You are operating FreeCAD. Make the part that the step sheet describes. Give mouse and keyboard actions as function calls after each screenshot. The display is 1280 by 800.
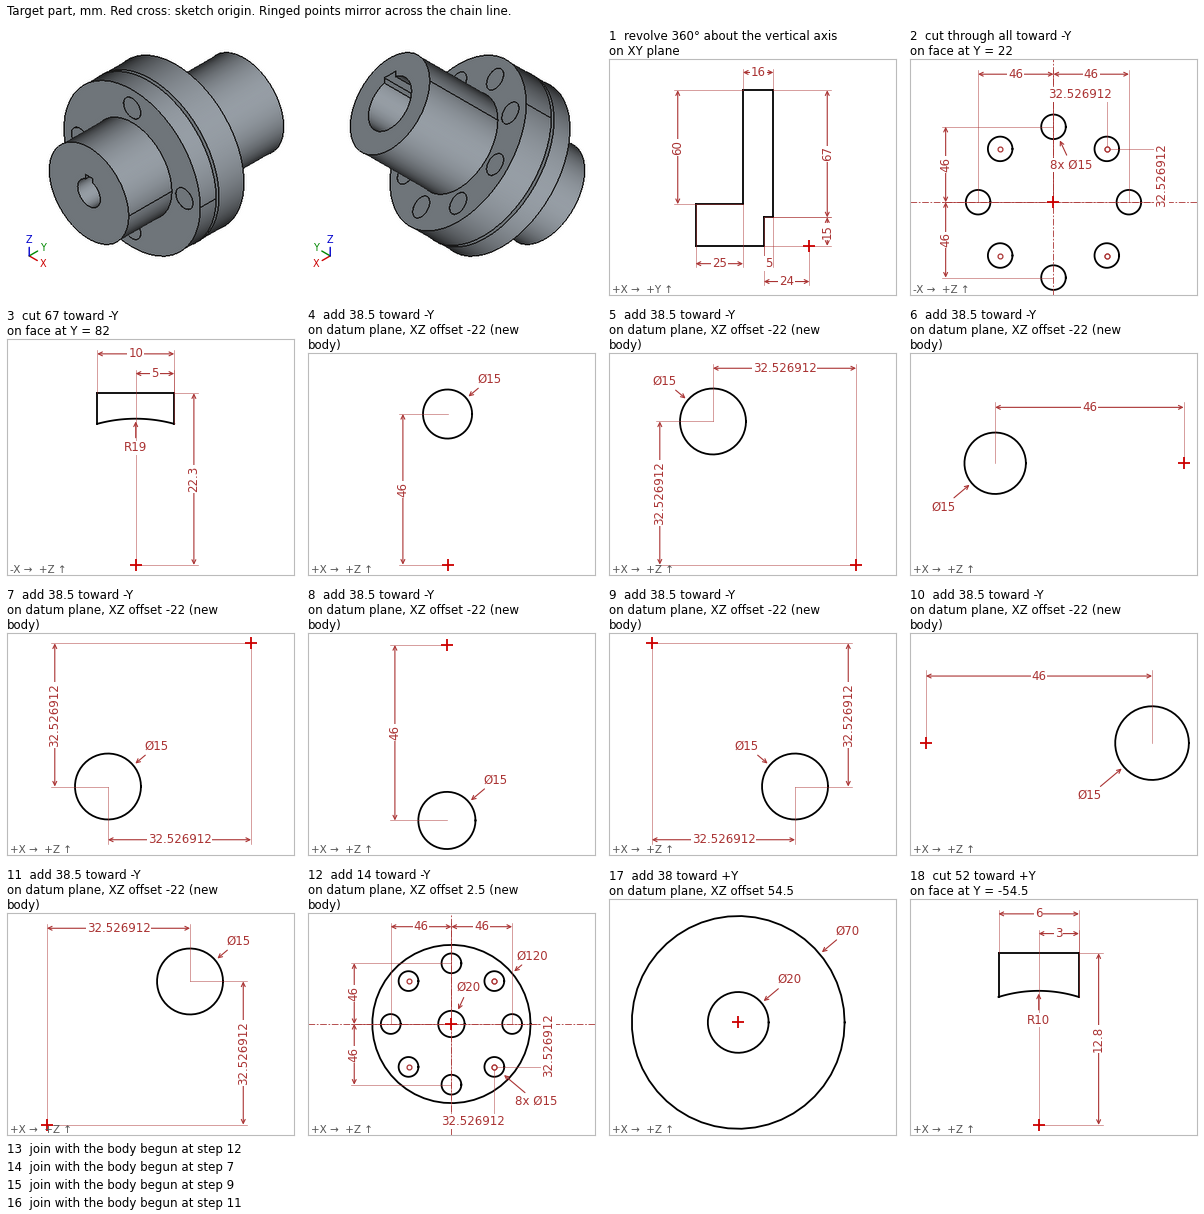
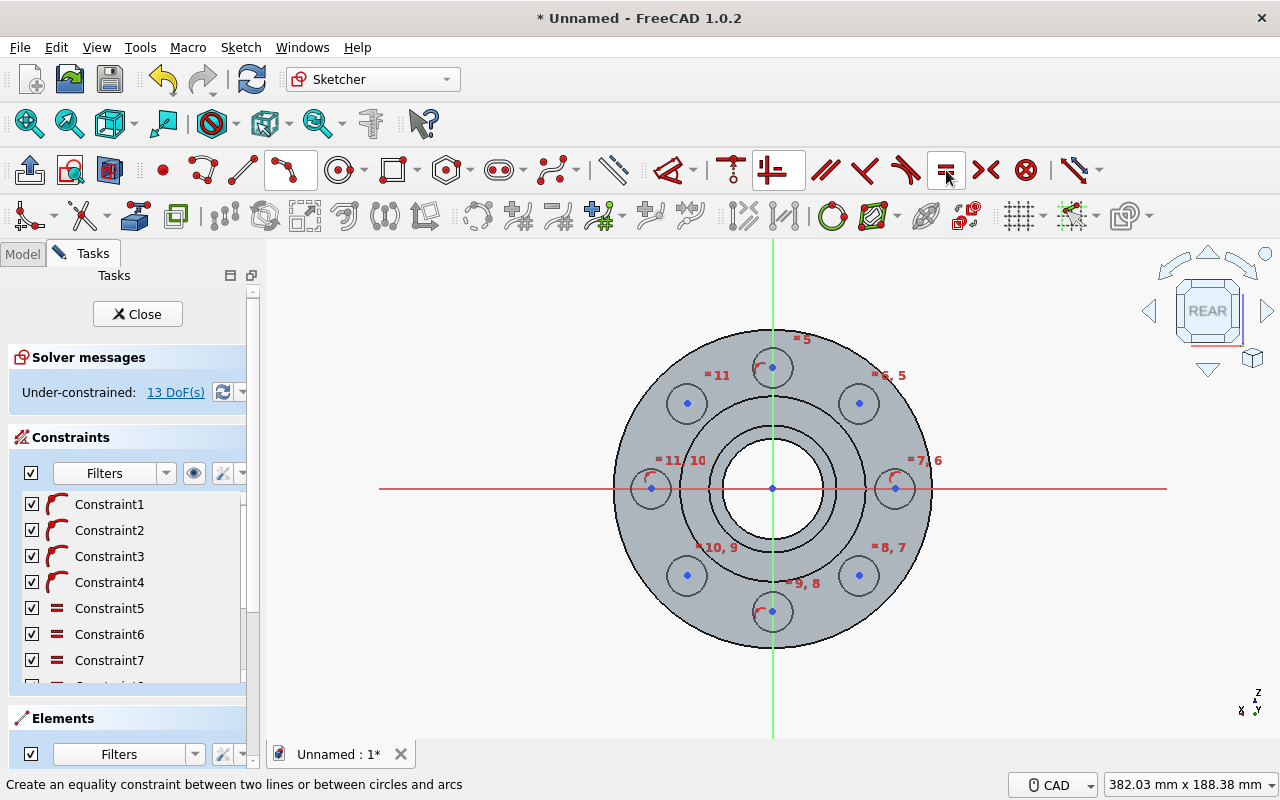
click(859, 404)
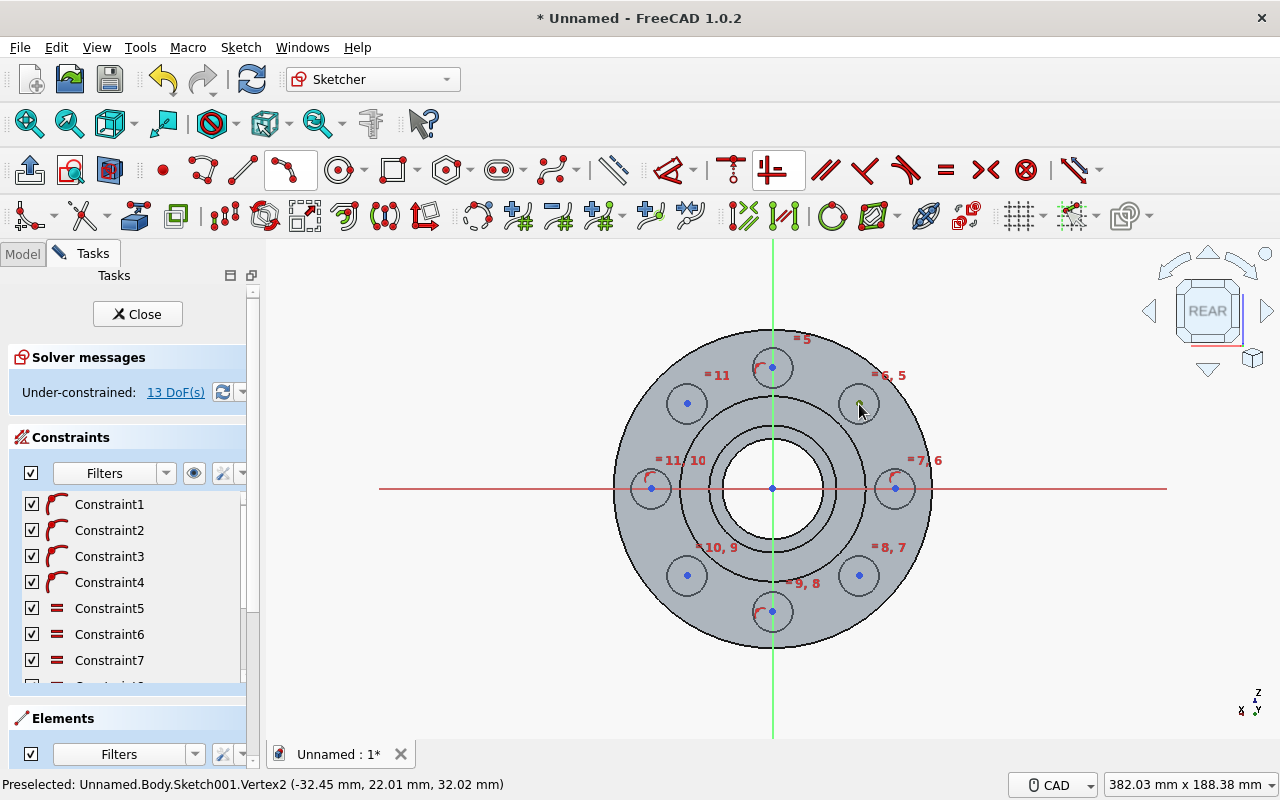
click(859, 576)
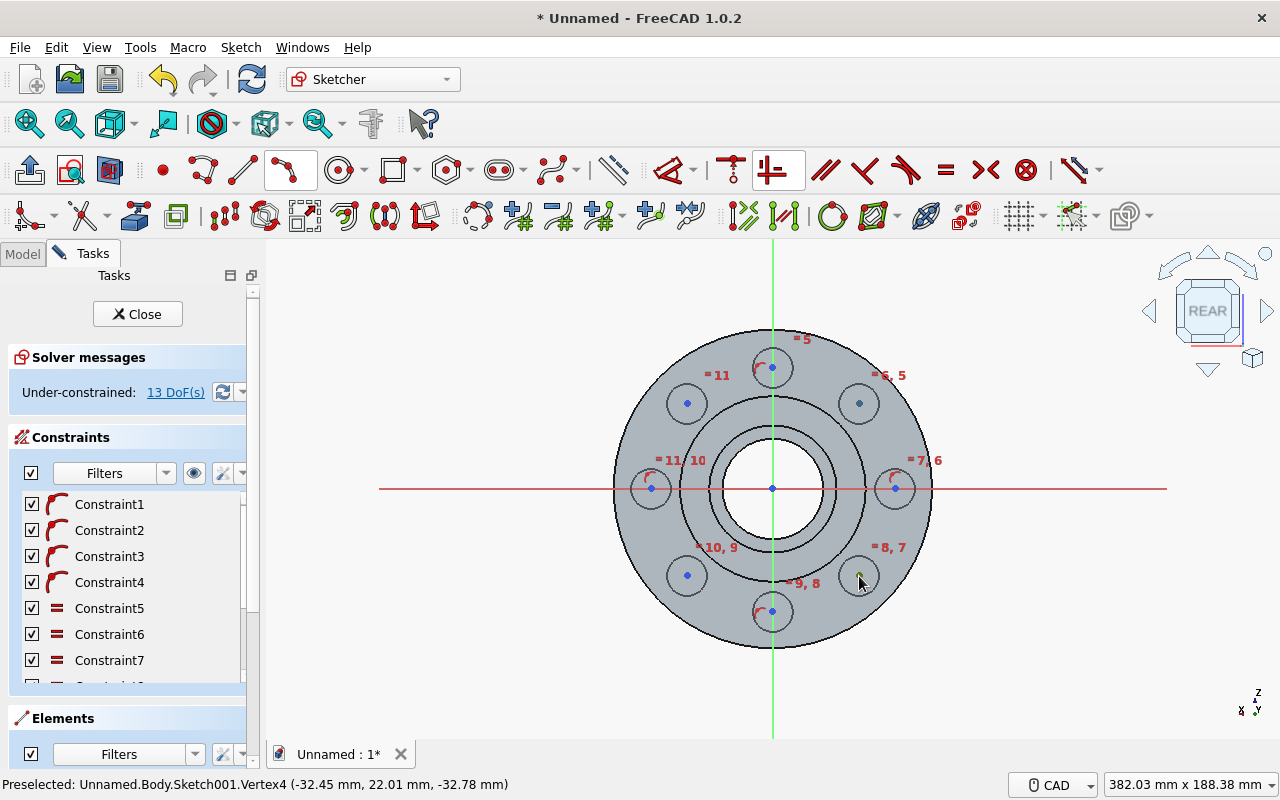
click(411, 489)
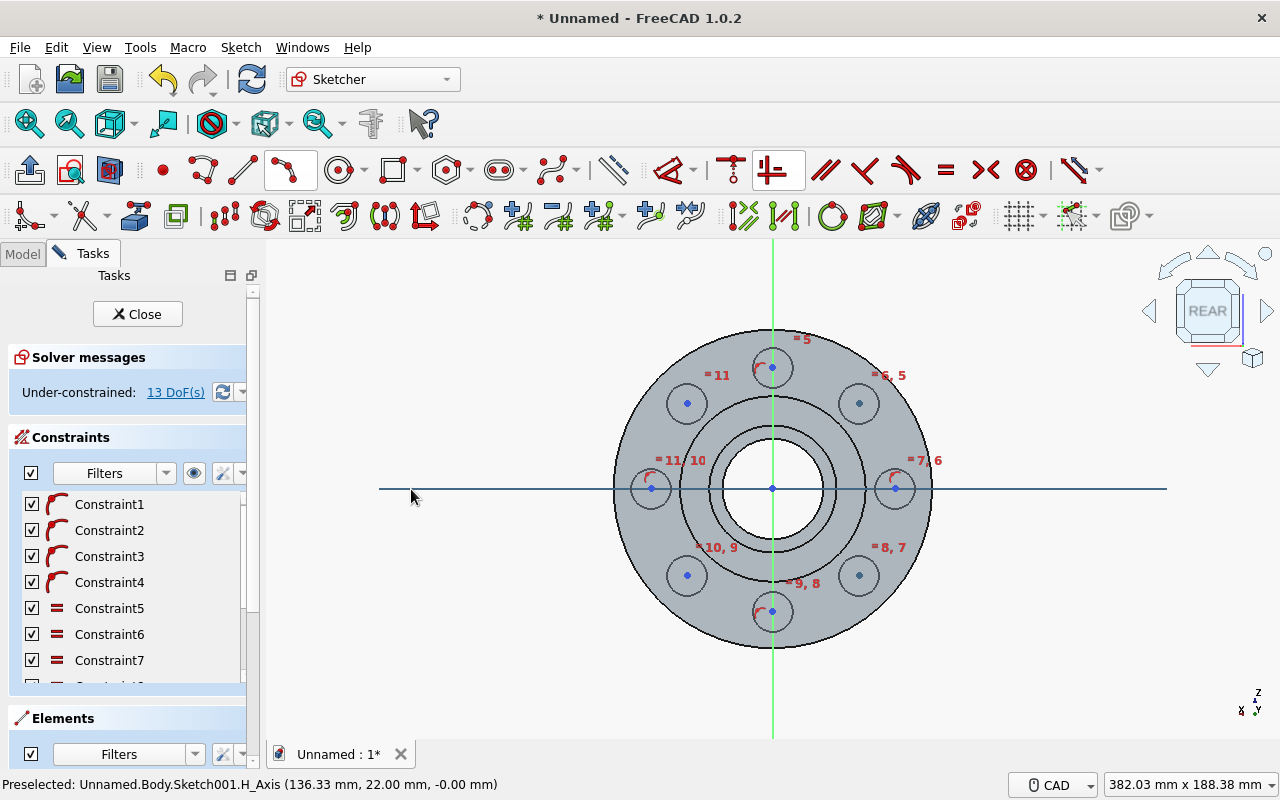
click(986, 170)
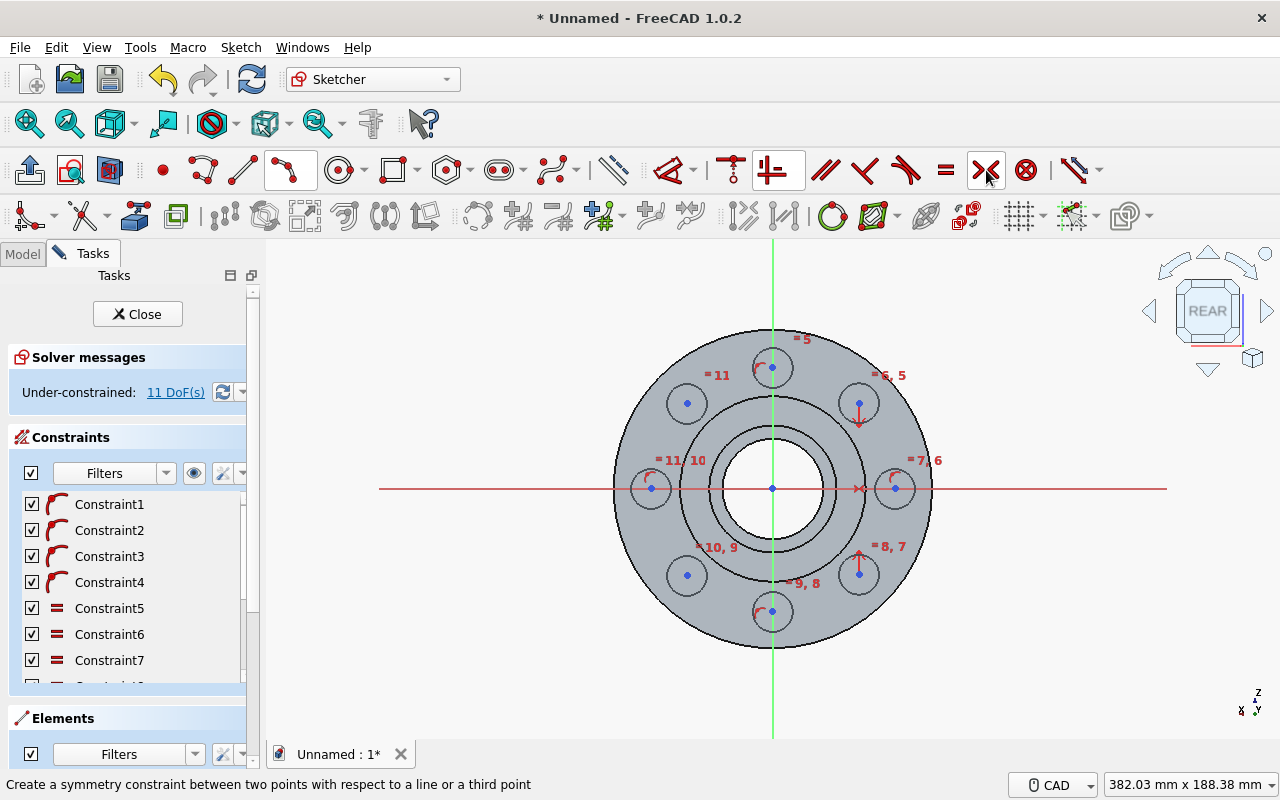
click(859, 575)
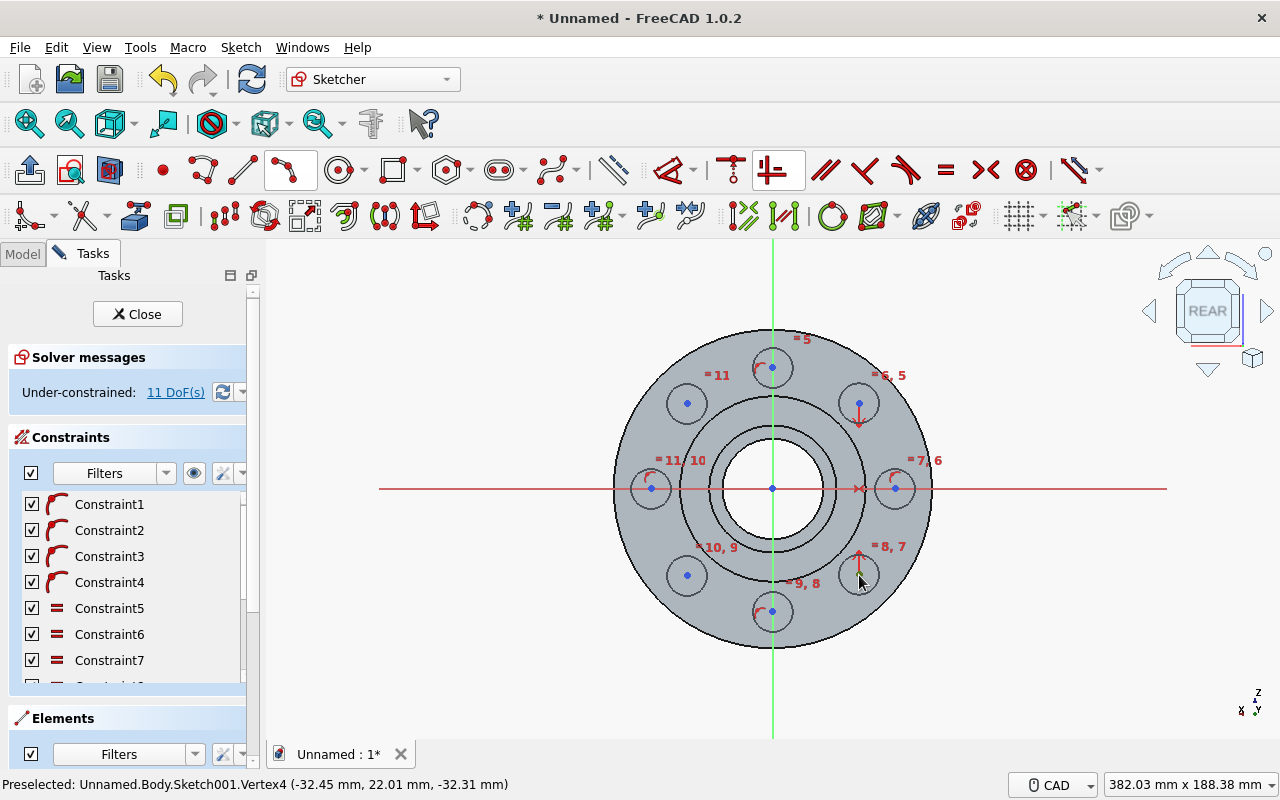
click(687, 576)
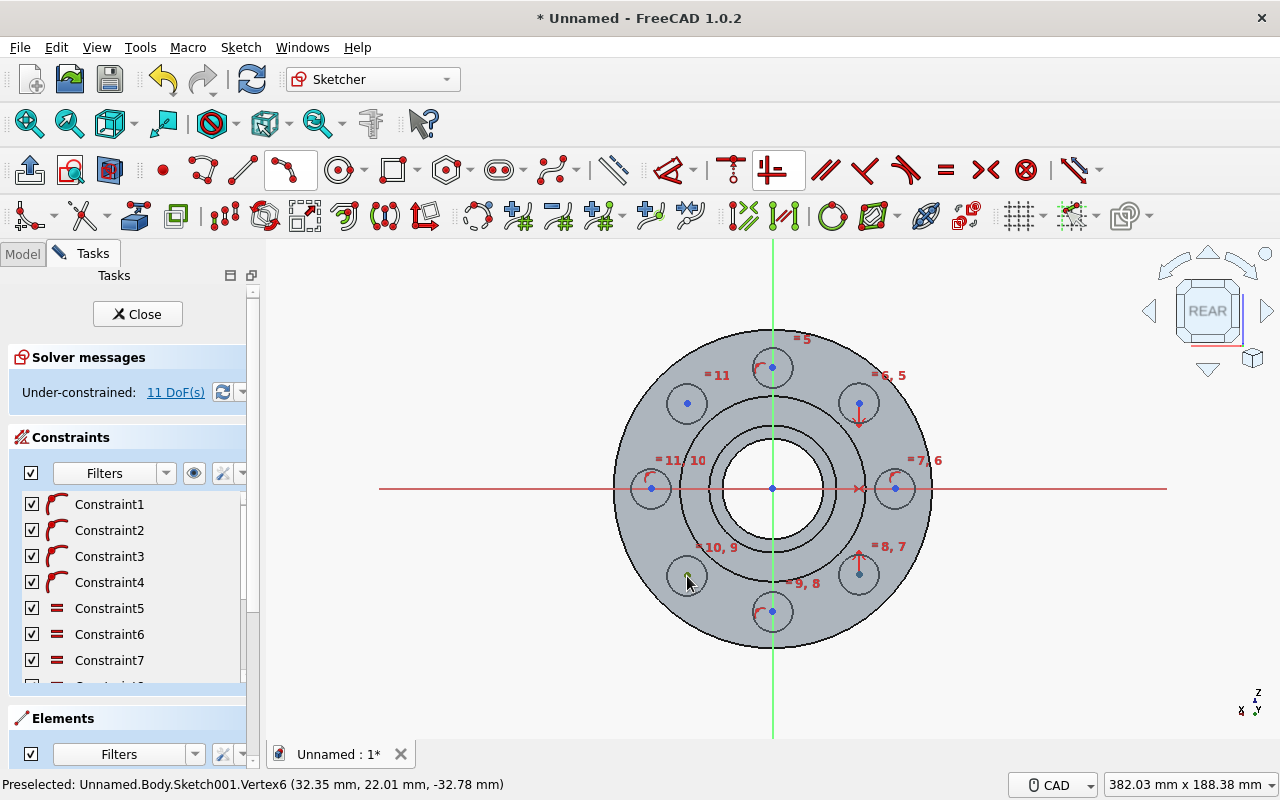
click(773, 679)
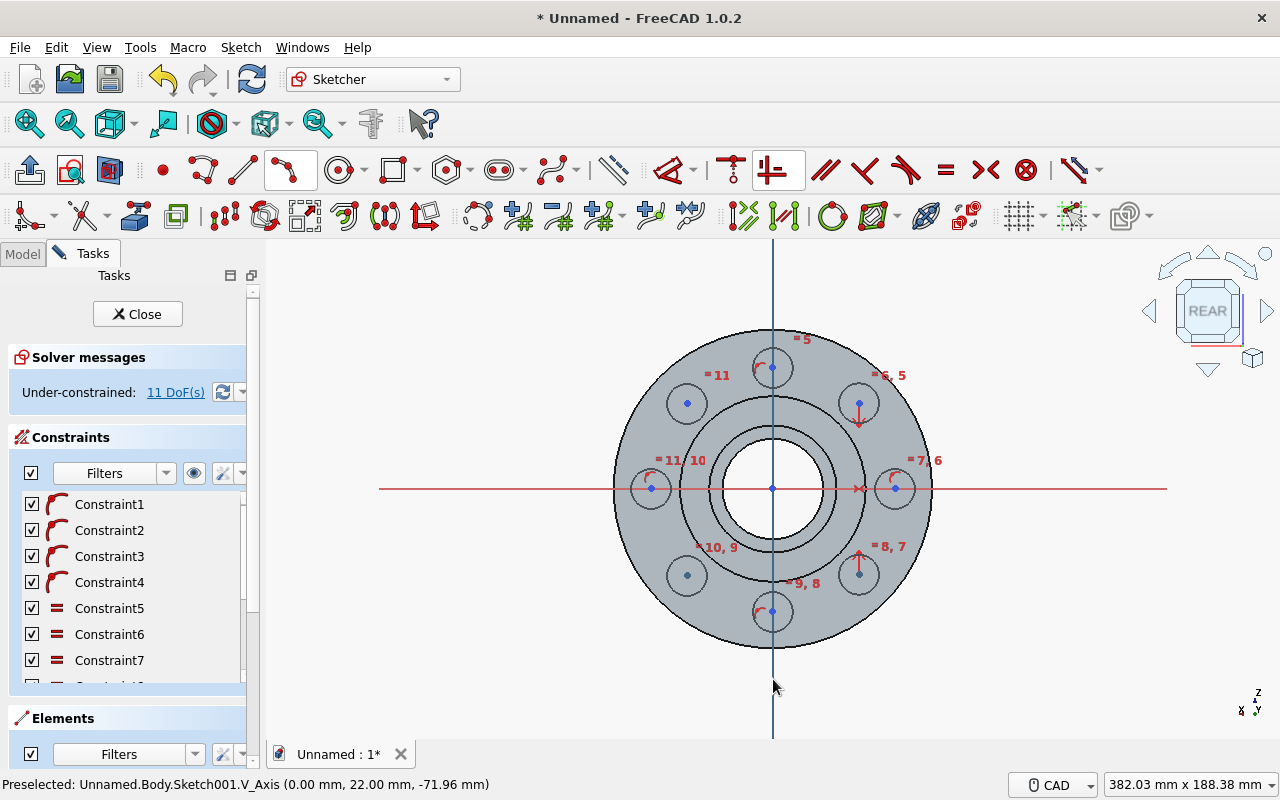
click(986, 170)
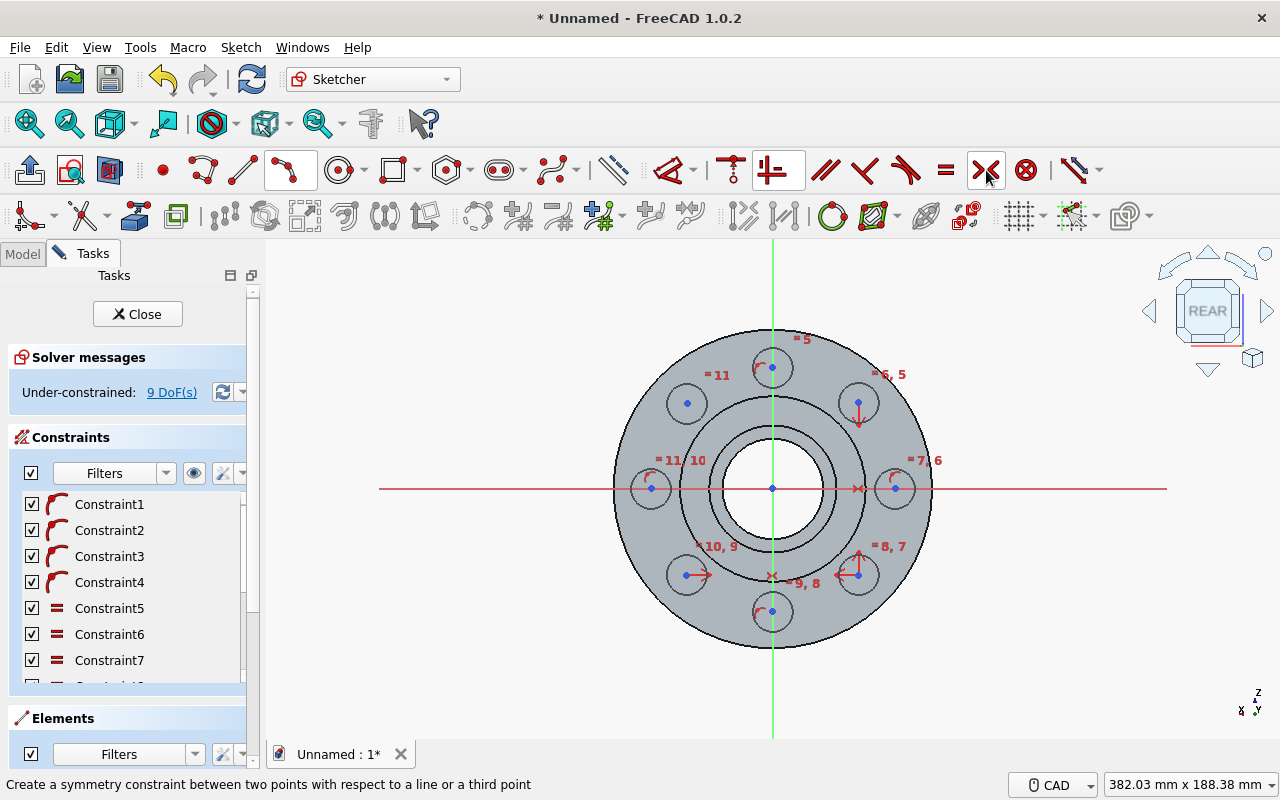
click(859, 403)